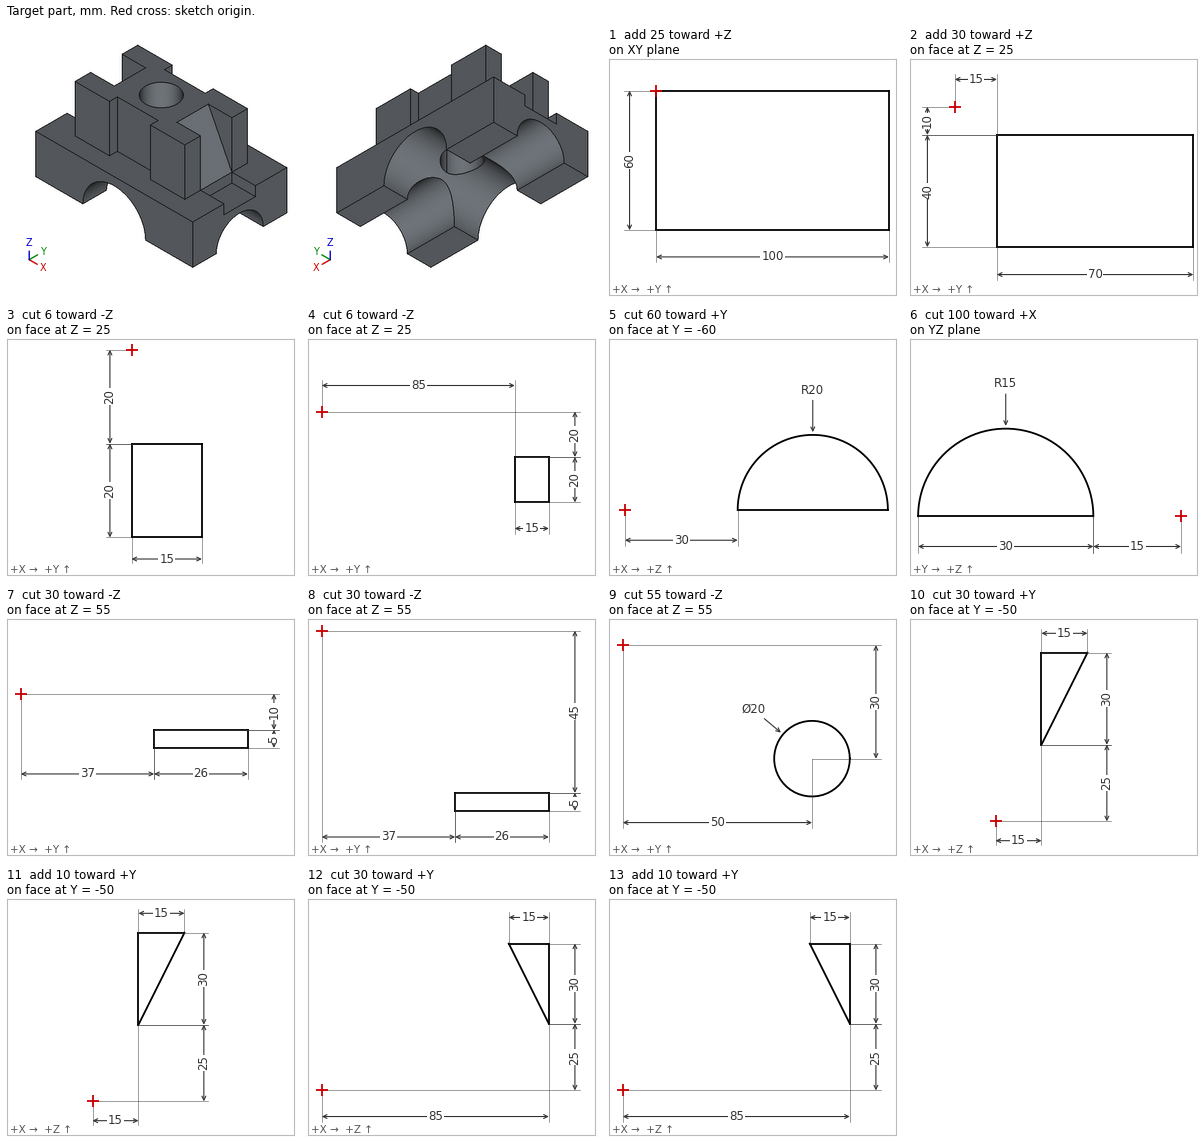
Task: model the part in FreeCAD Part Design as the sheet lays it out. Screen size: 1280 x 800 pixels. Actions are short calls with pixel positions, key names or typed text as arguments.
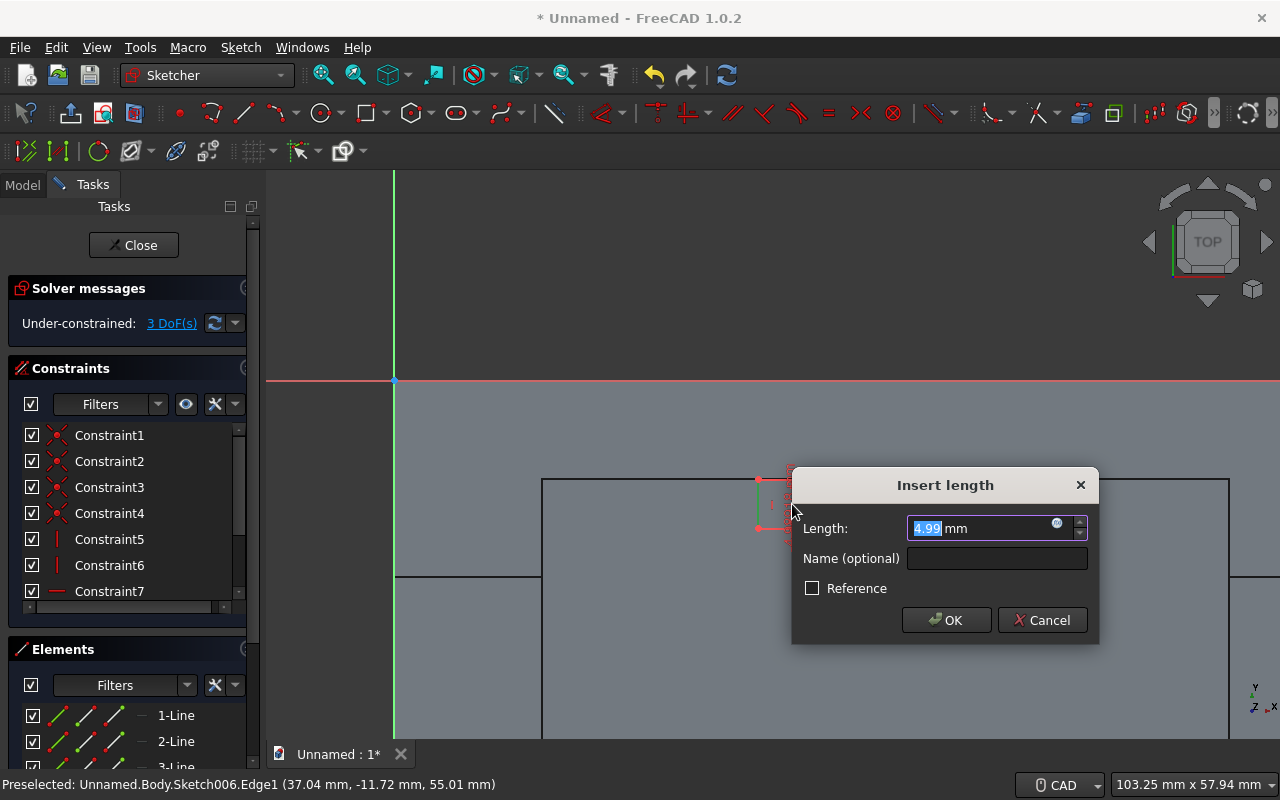
text(5)
key(Return)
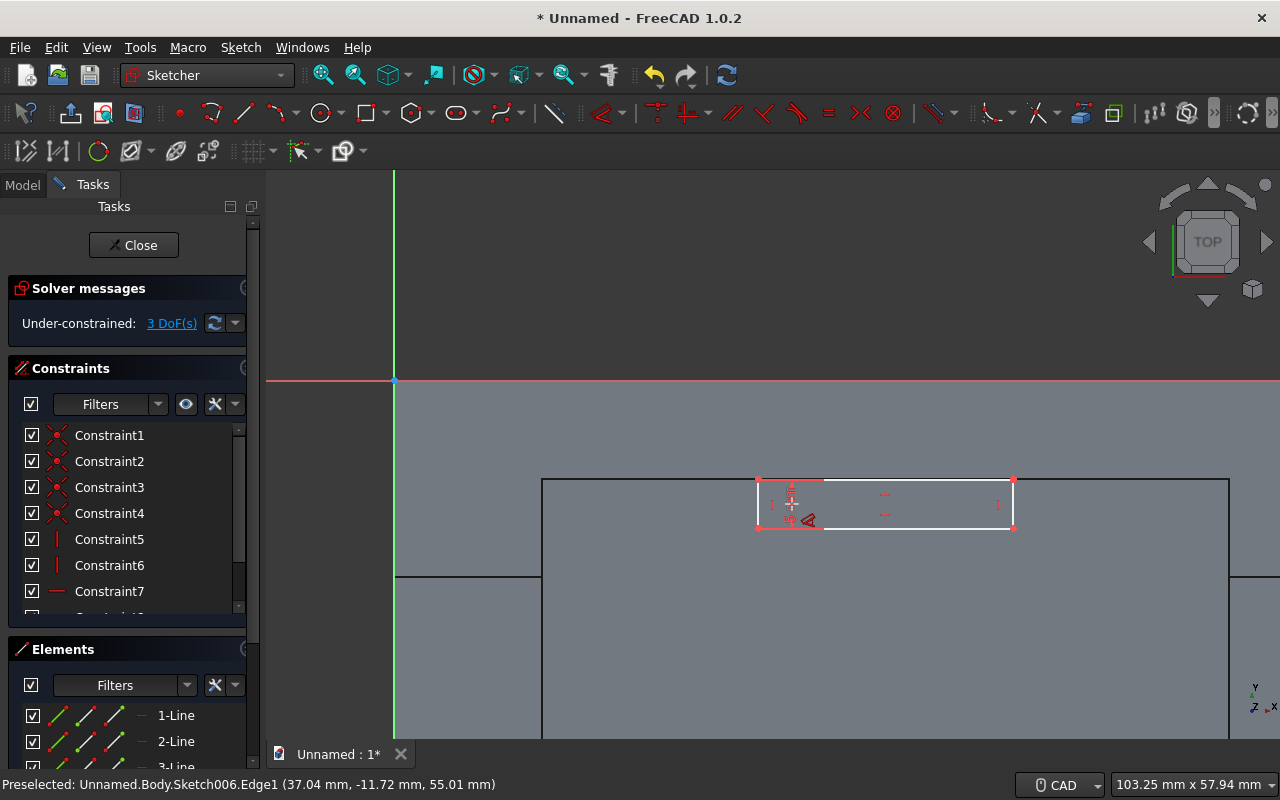
click(835, 529)
click(885, 563)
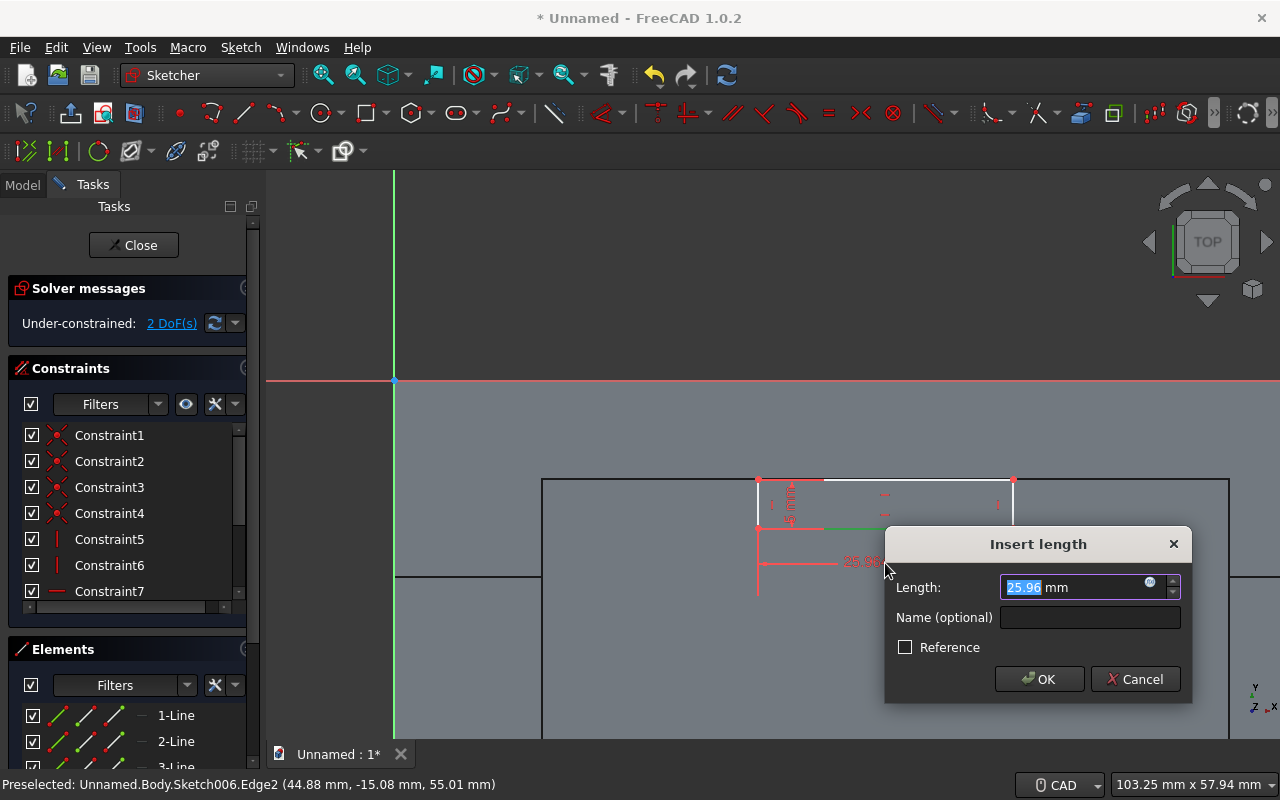
text(26)
key(Return)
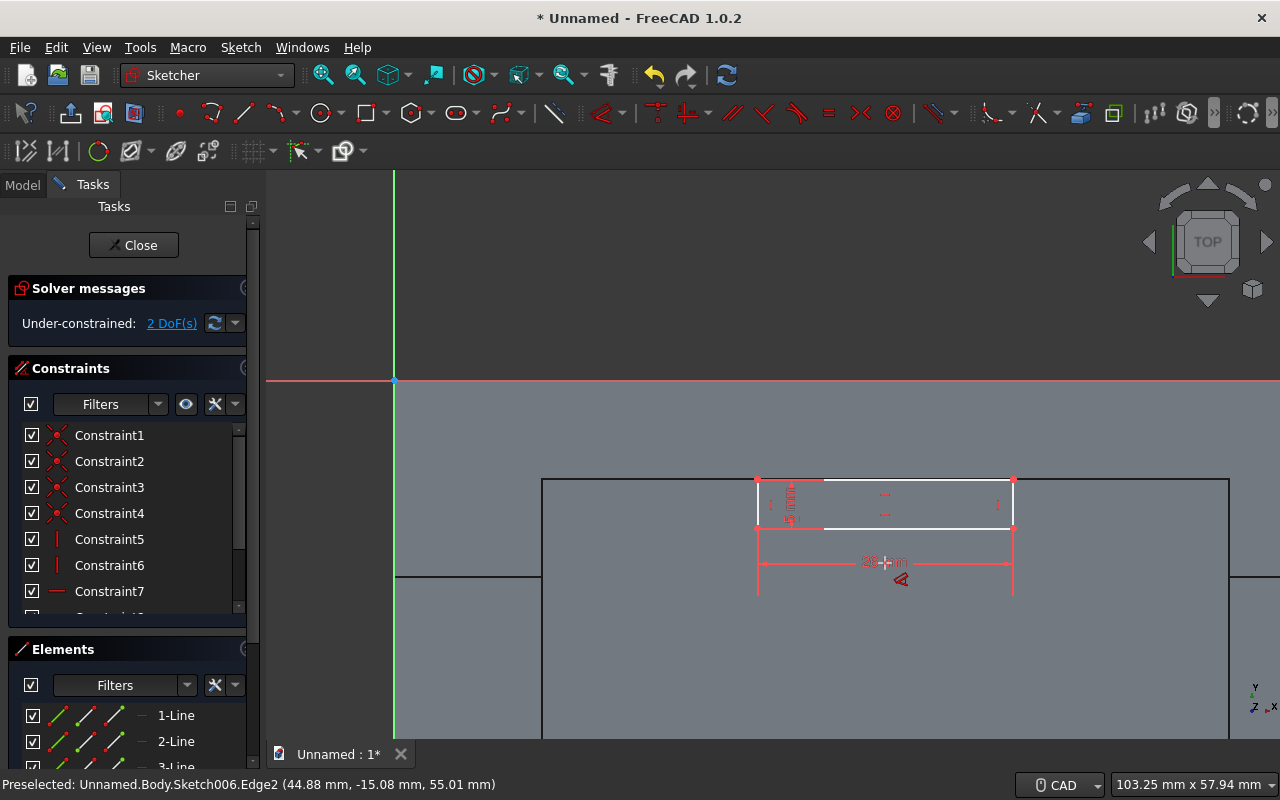
click(758, 480)
click(576, 347)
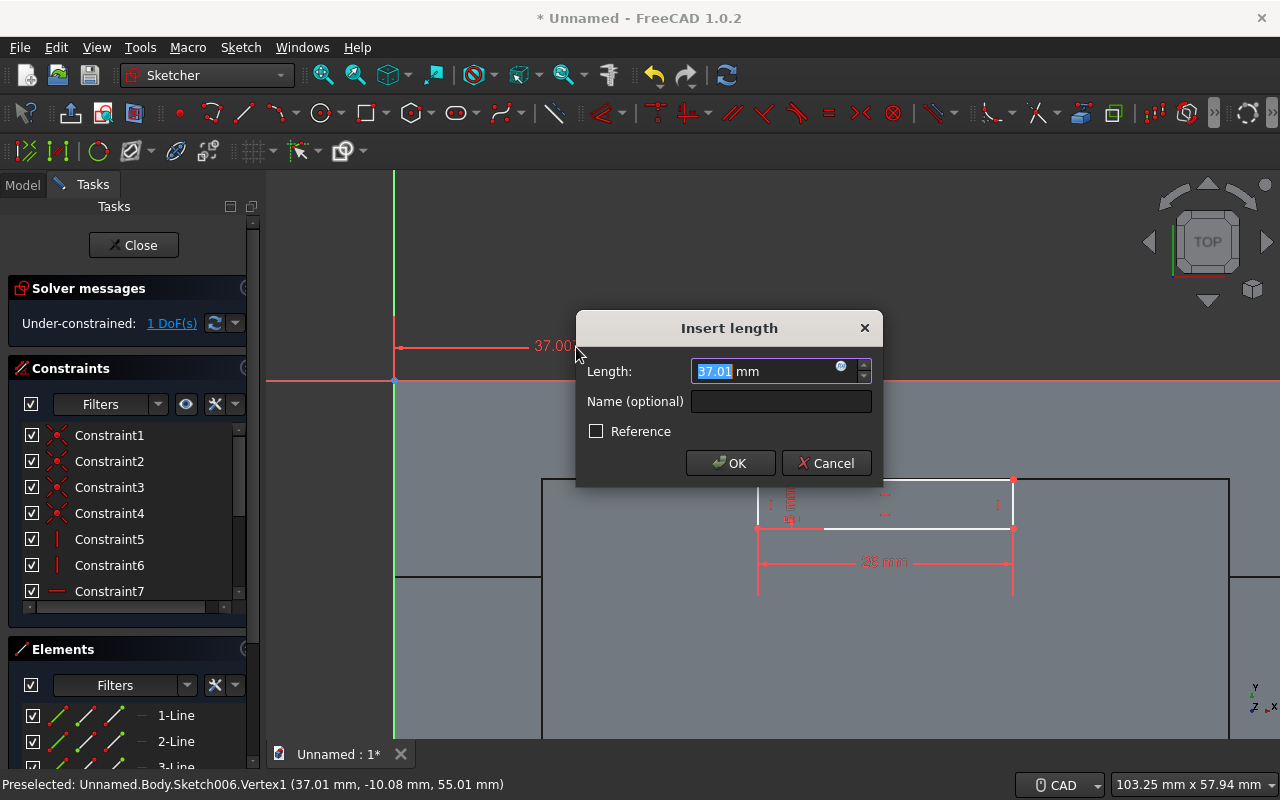
text(37)
key(Return)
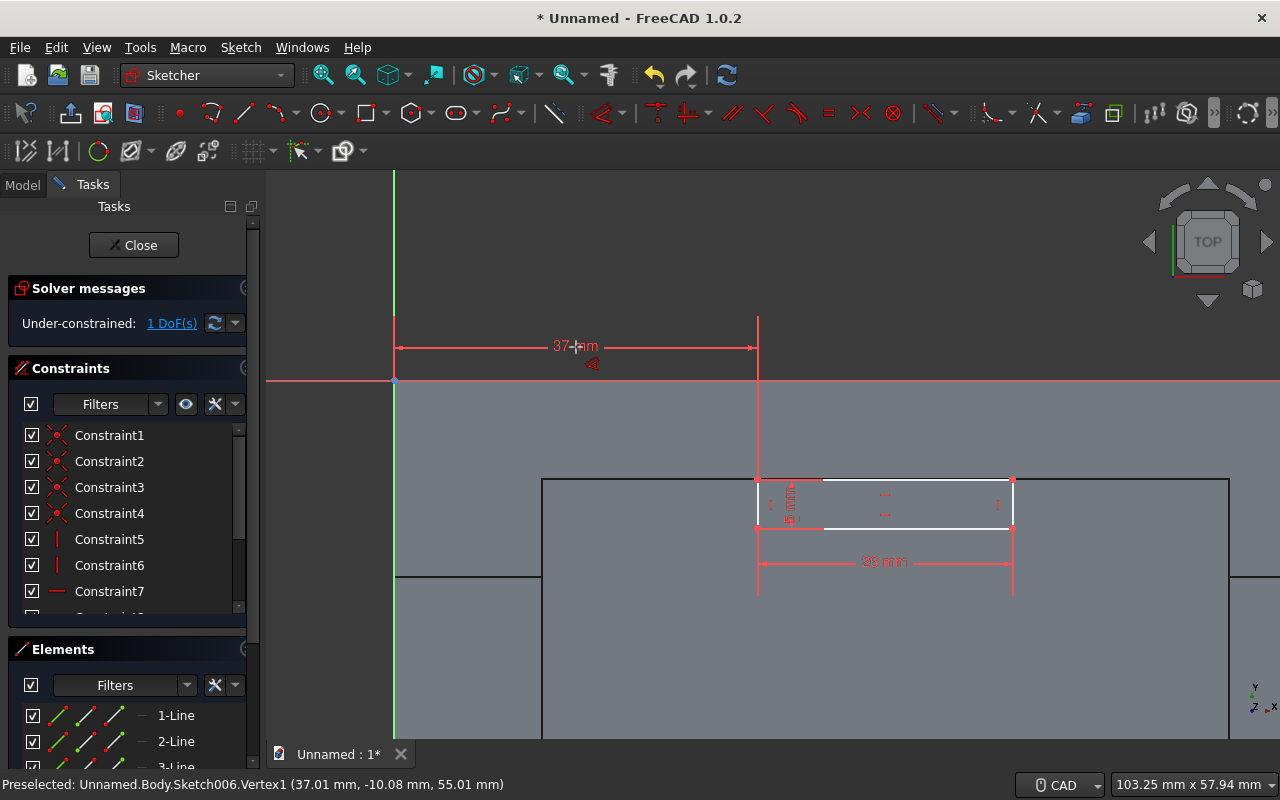
click(758, 480)
click(360, 430)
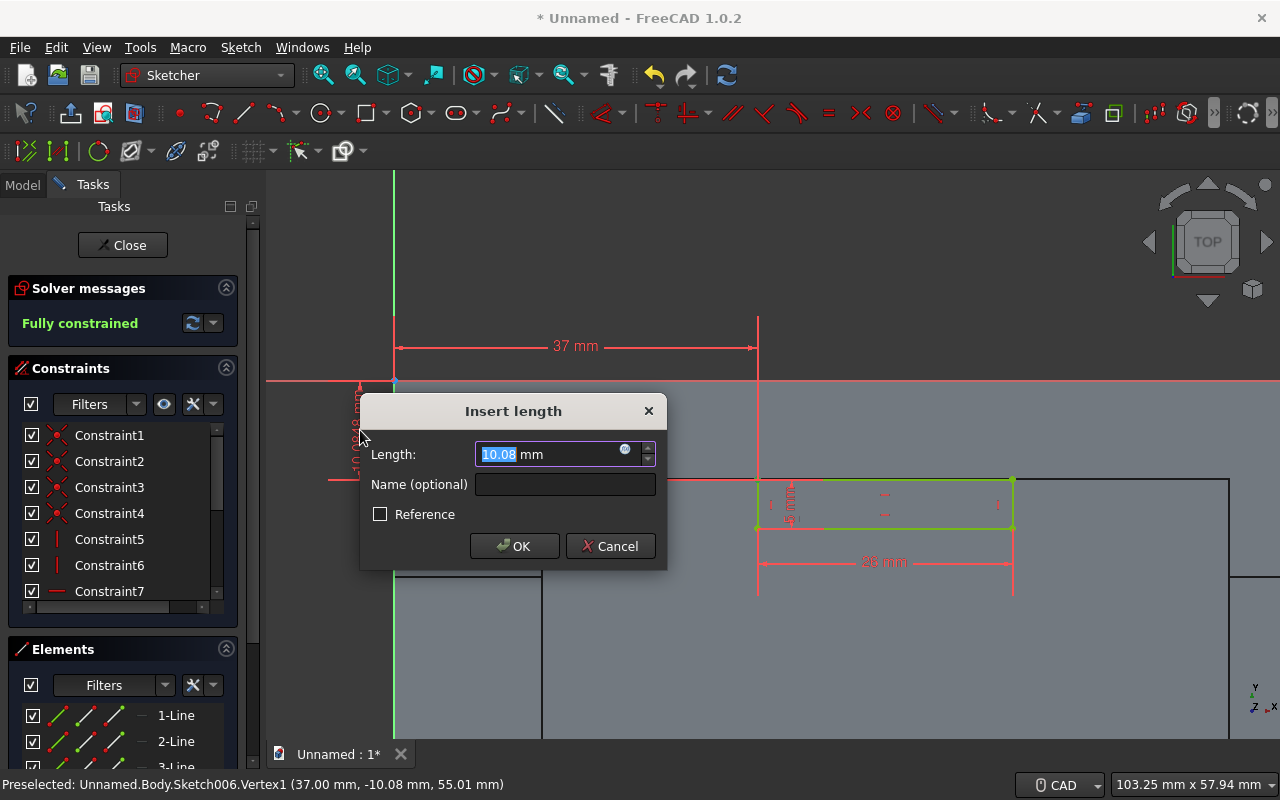
text(10)
key(Return)
key(Escape)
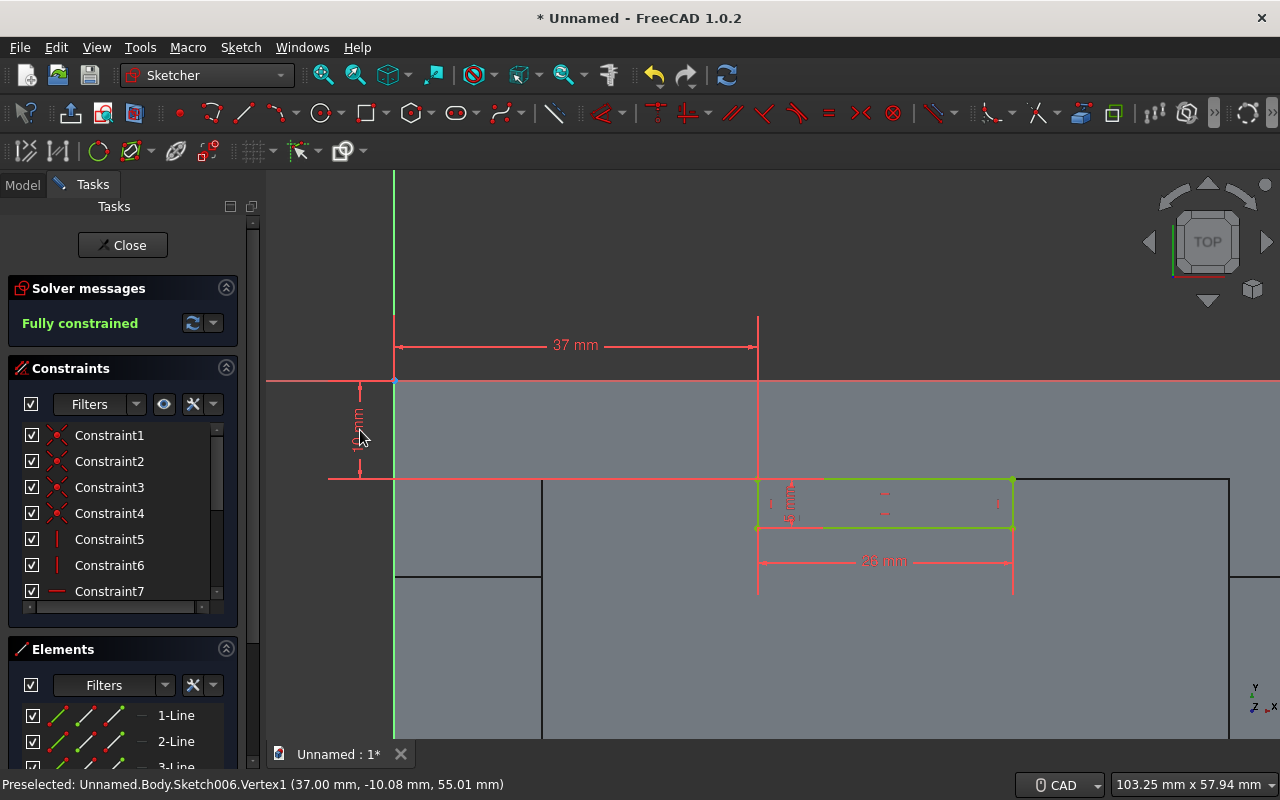
click(123, 245)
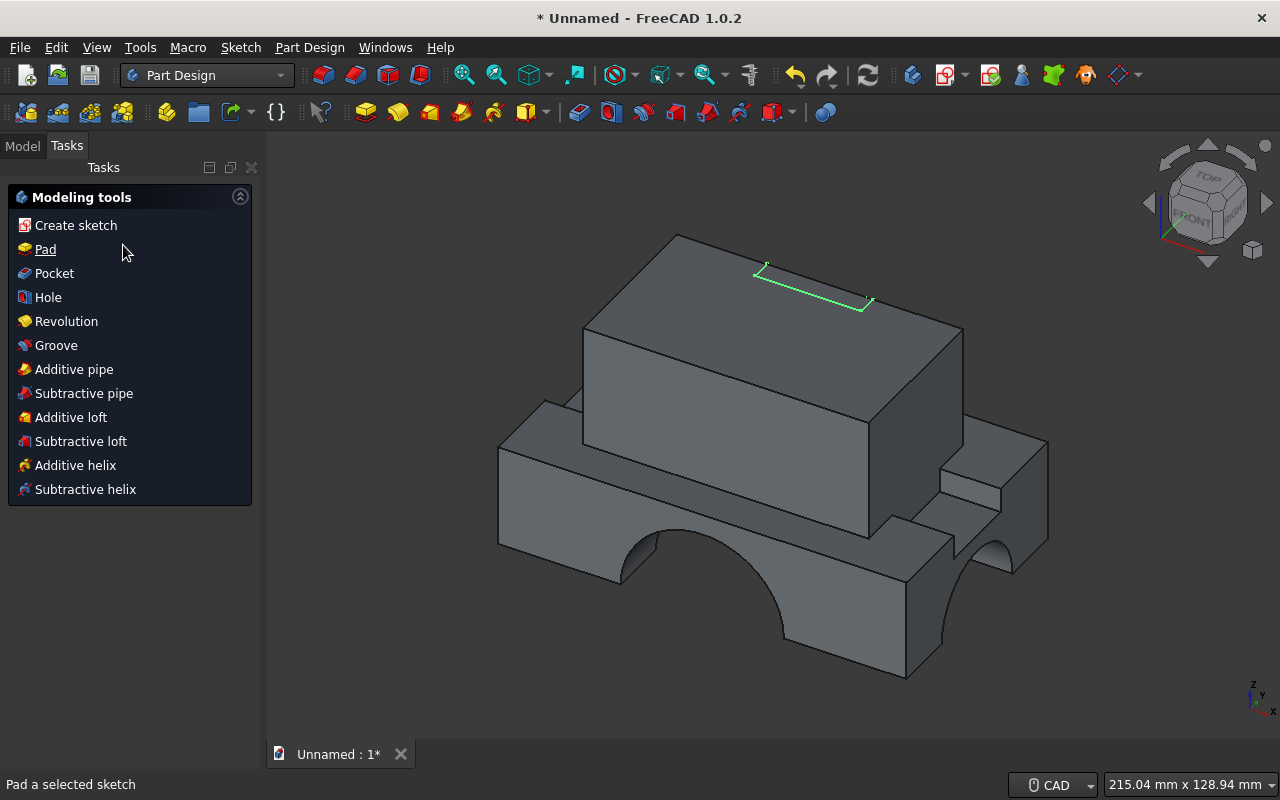
click(580, 112)